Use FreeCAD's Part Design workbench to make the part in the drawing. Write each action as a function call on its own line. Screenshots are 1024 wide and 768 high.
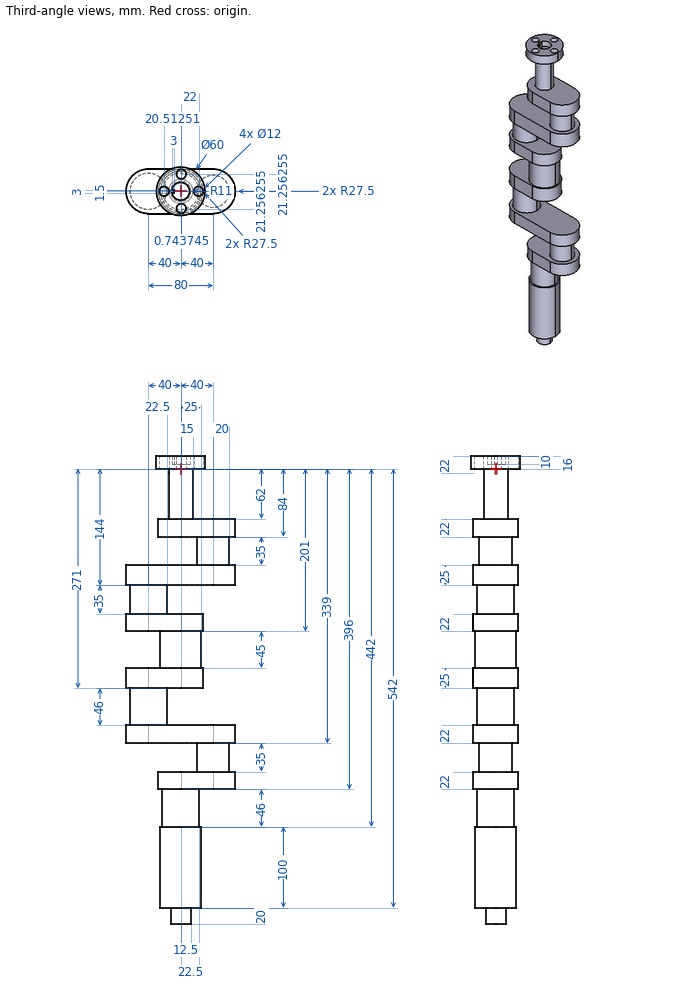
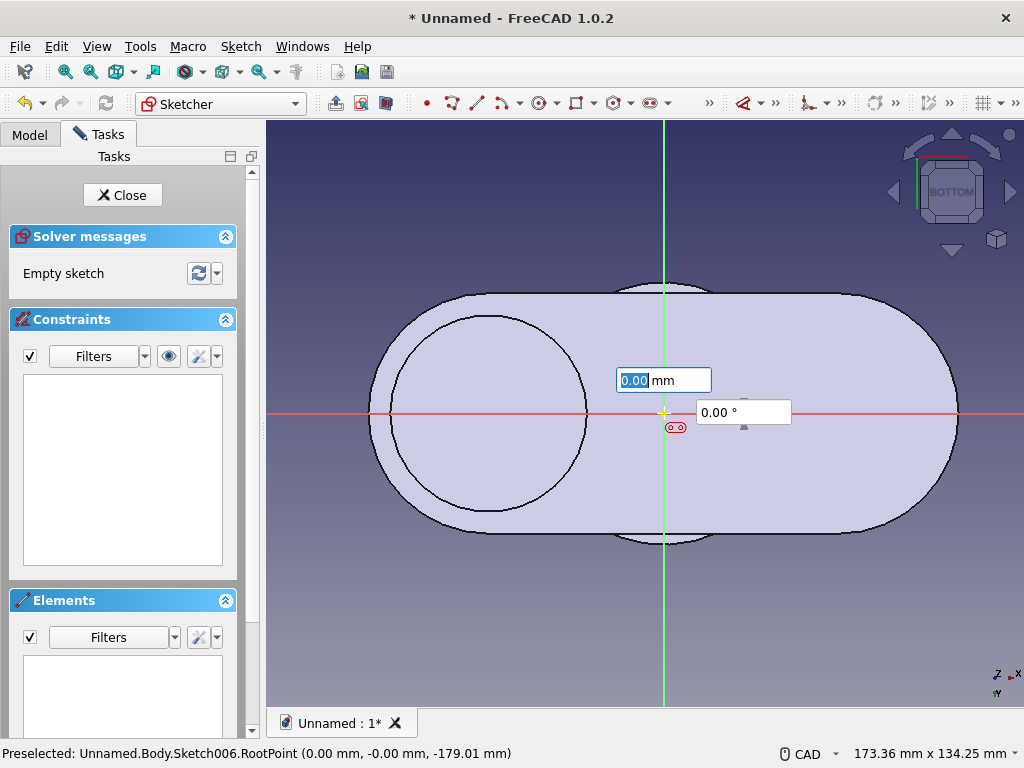
click(489, 404)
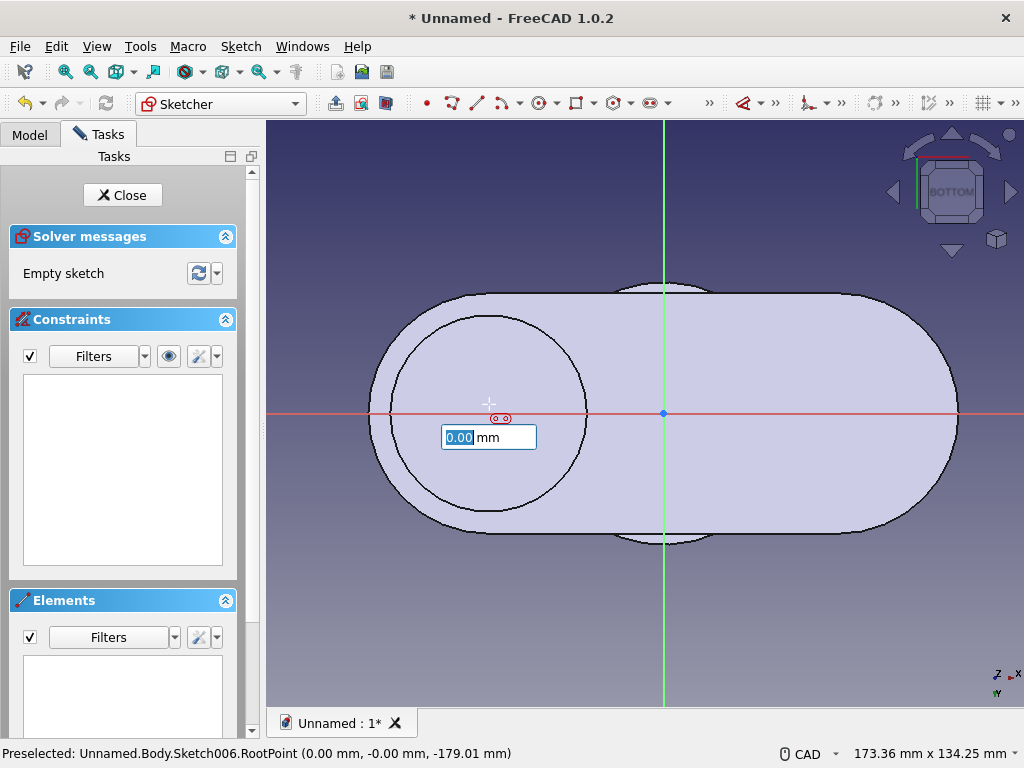
click(576, 534)
key(Escape)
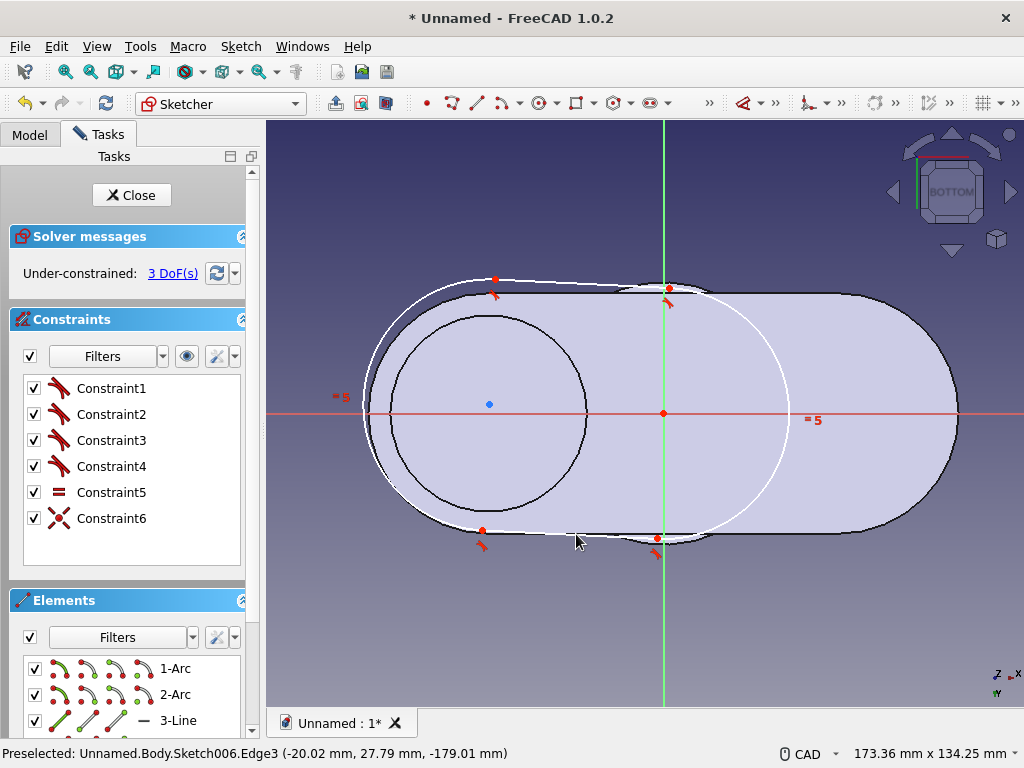
click(605, 536)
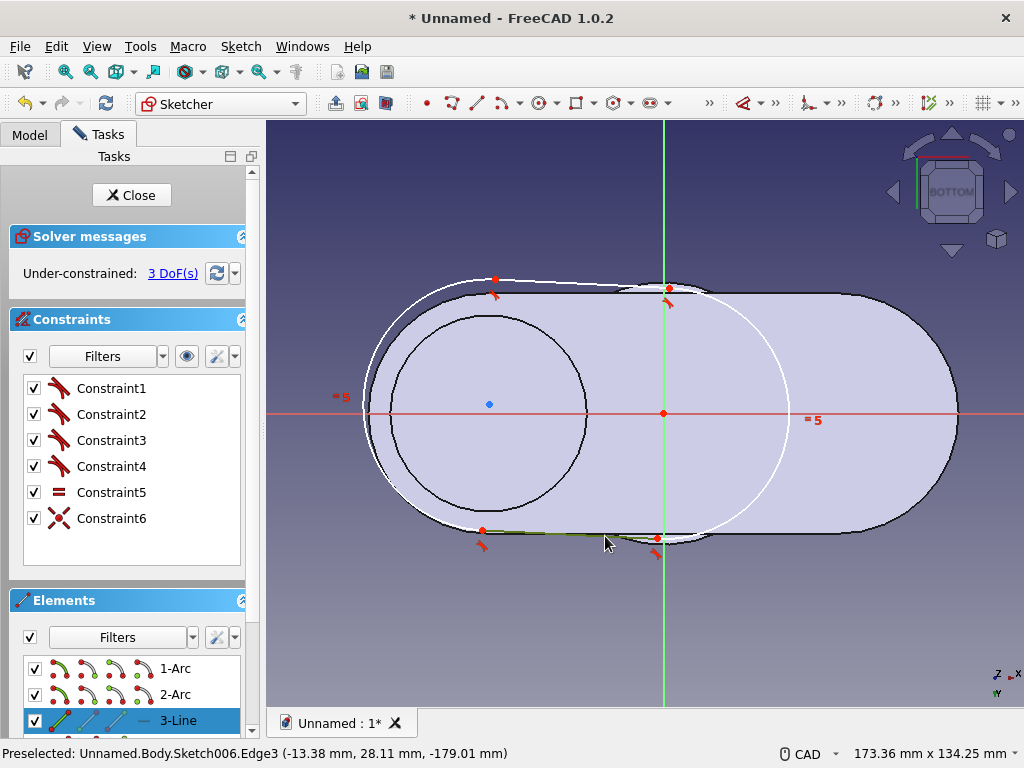
key(h)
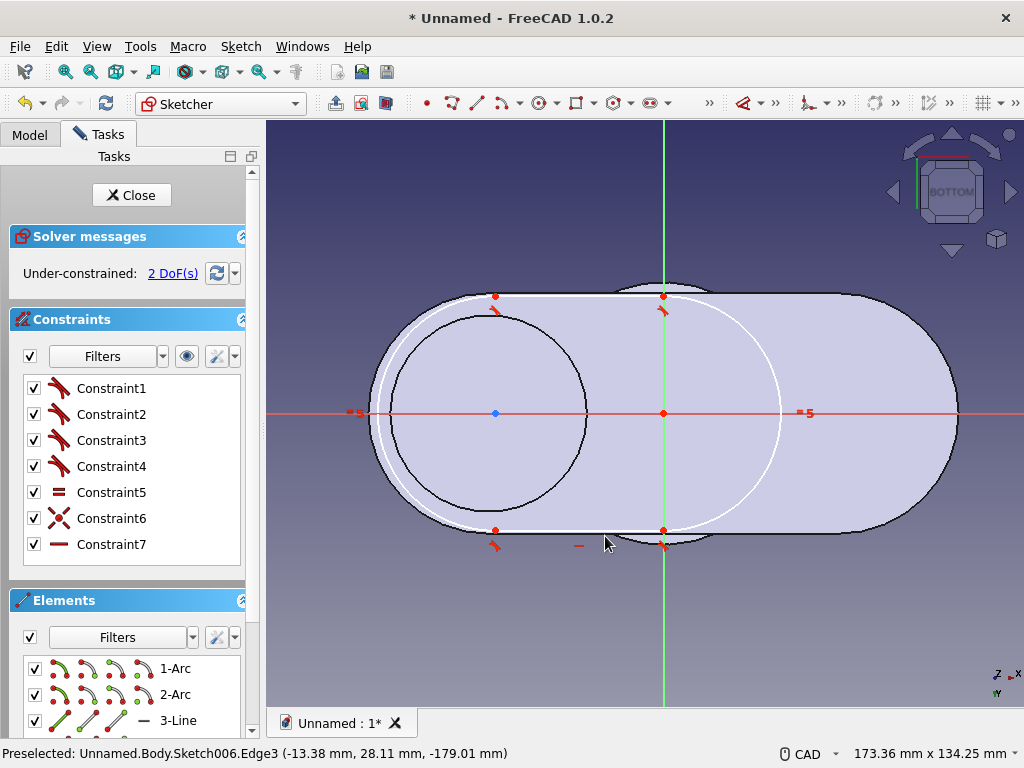
click(742, 104)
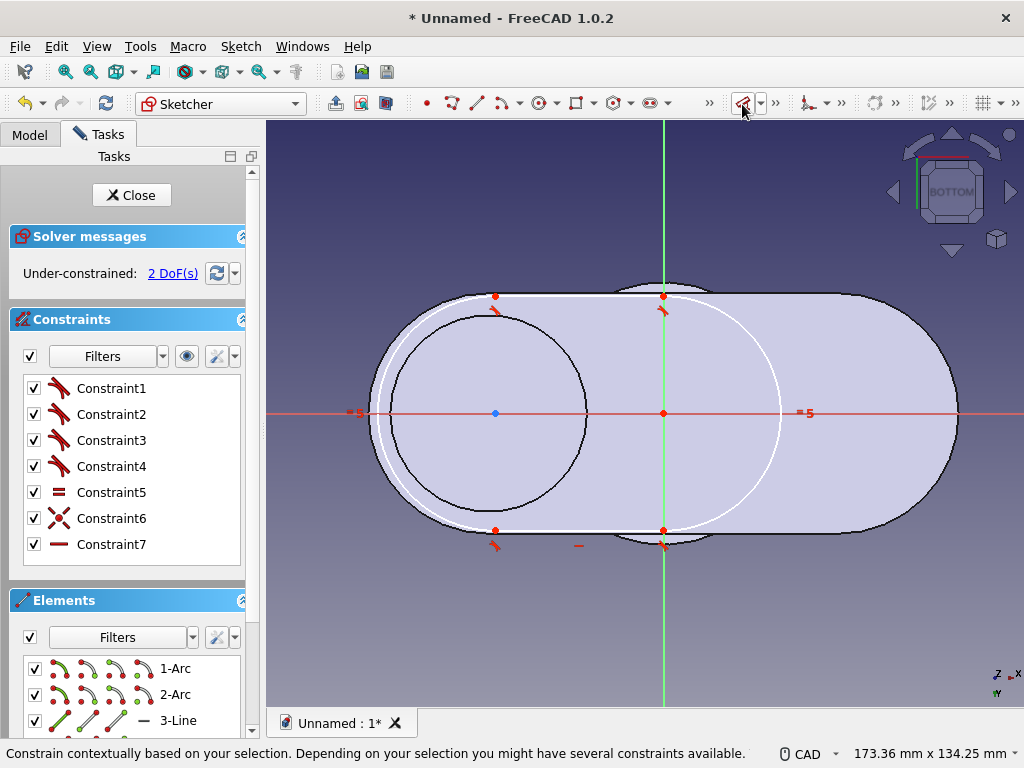
click(758, 482)
click(784, 501)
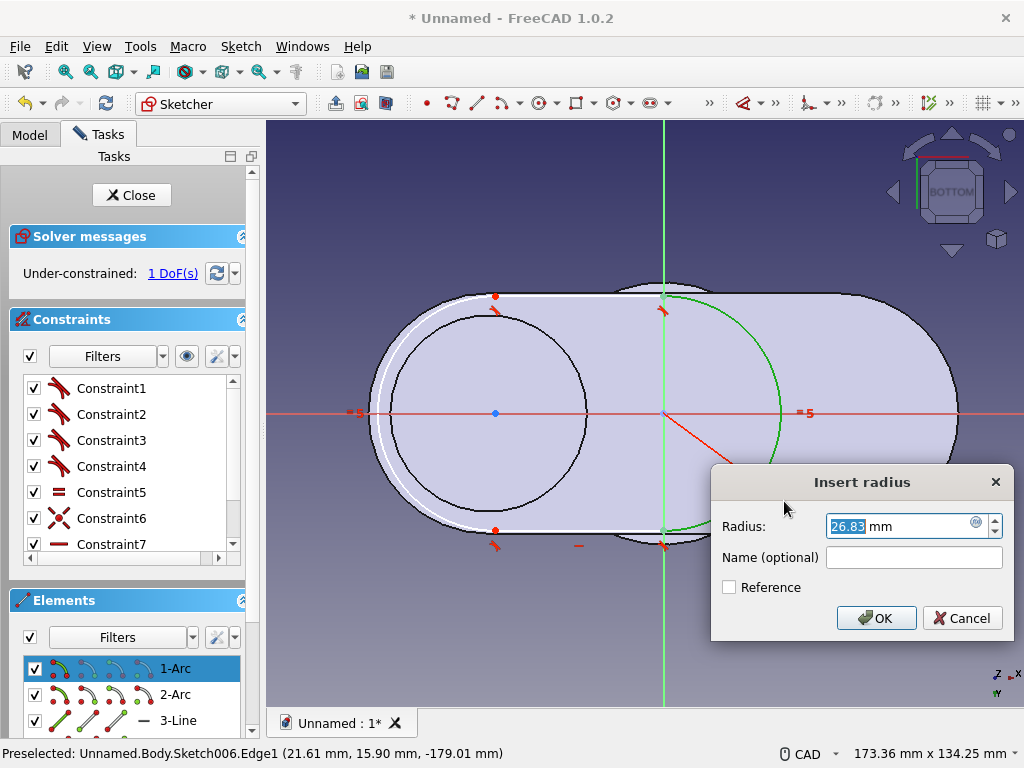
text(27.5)
key(Return)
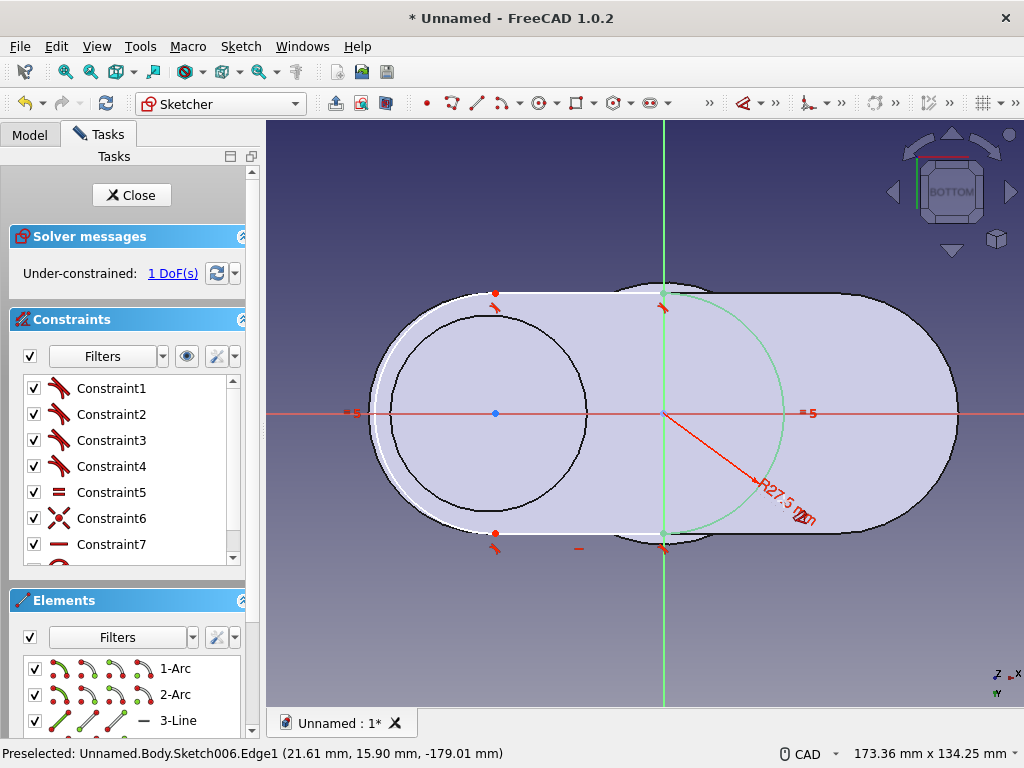
click(613, 534)
click(579, 568)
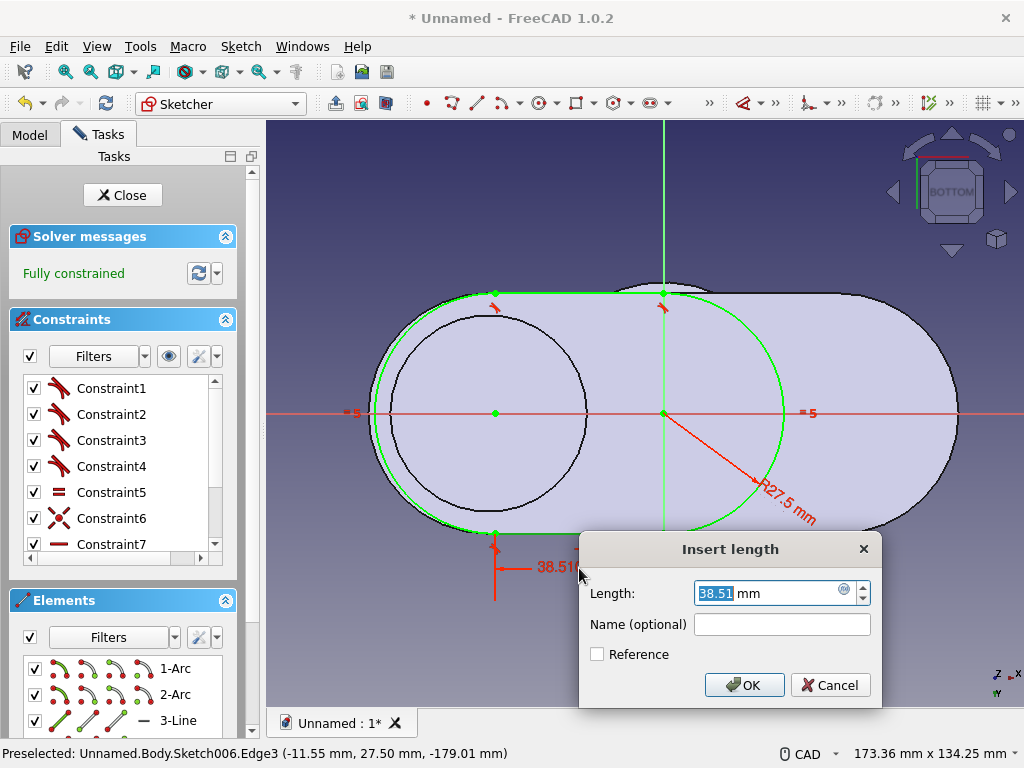
text(40)
key(Return)
key(Escape)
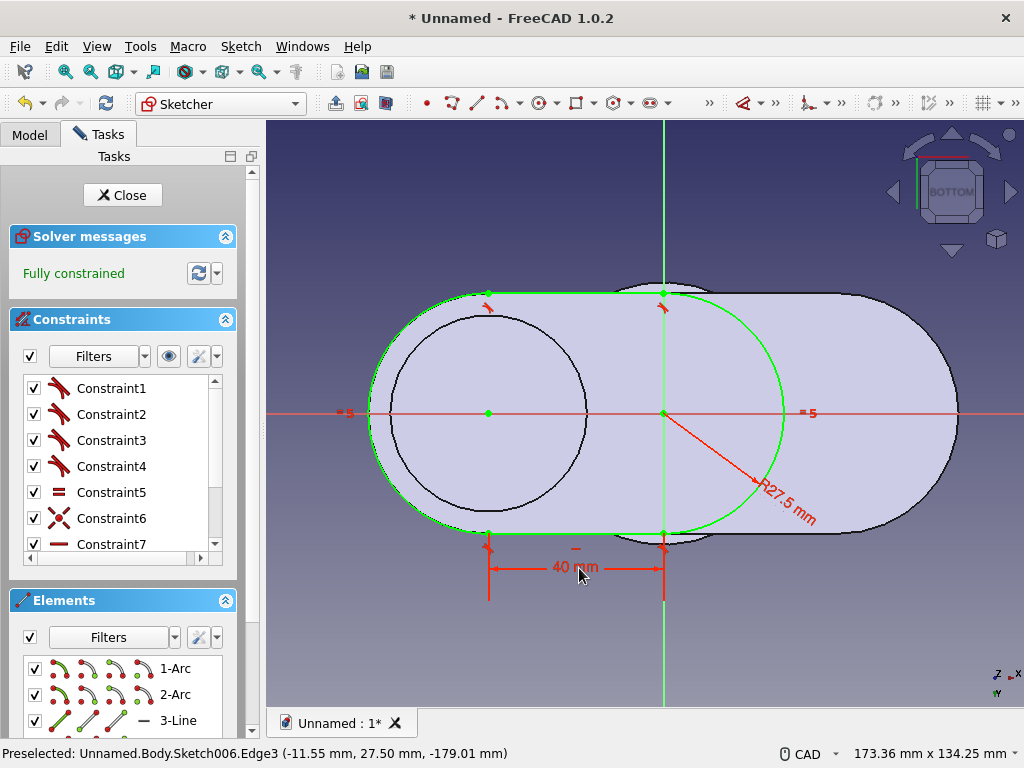
click(123, 195)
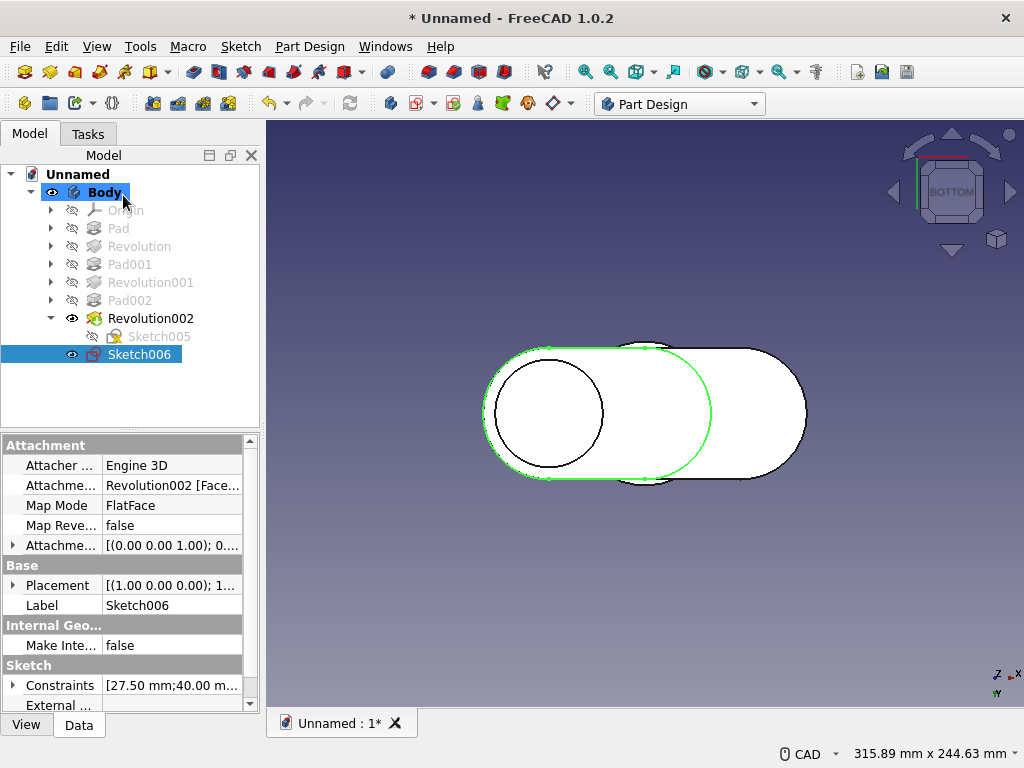
click(25, 72)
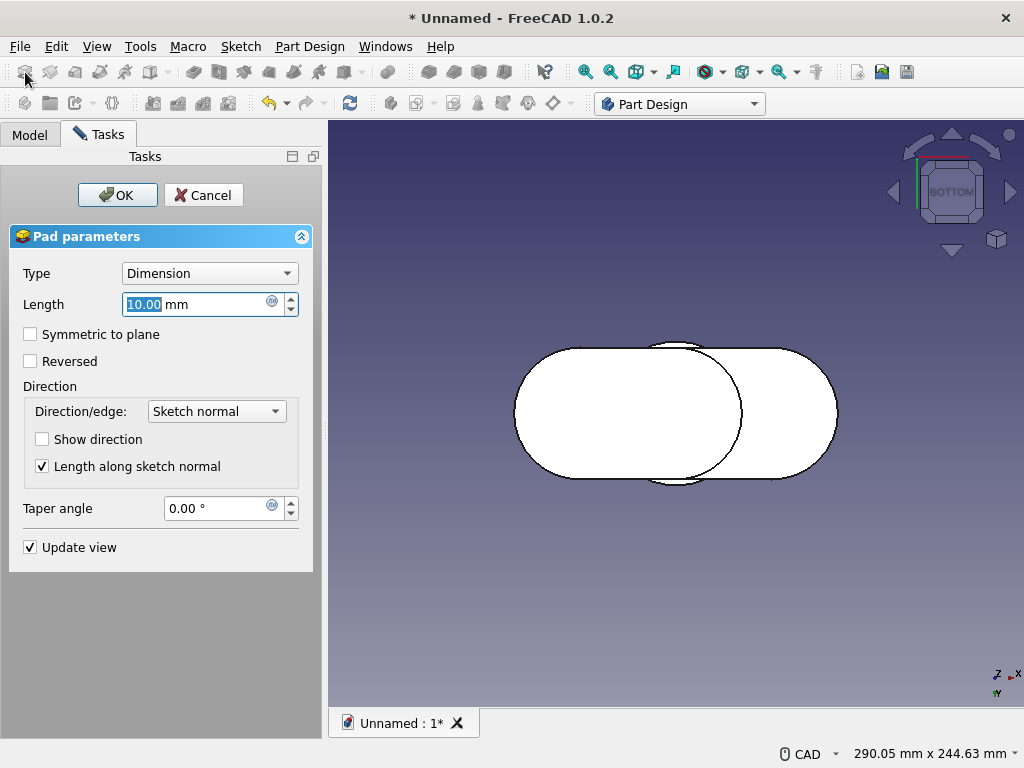
text(22)
key(Tab)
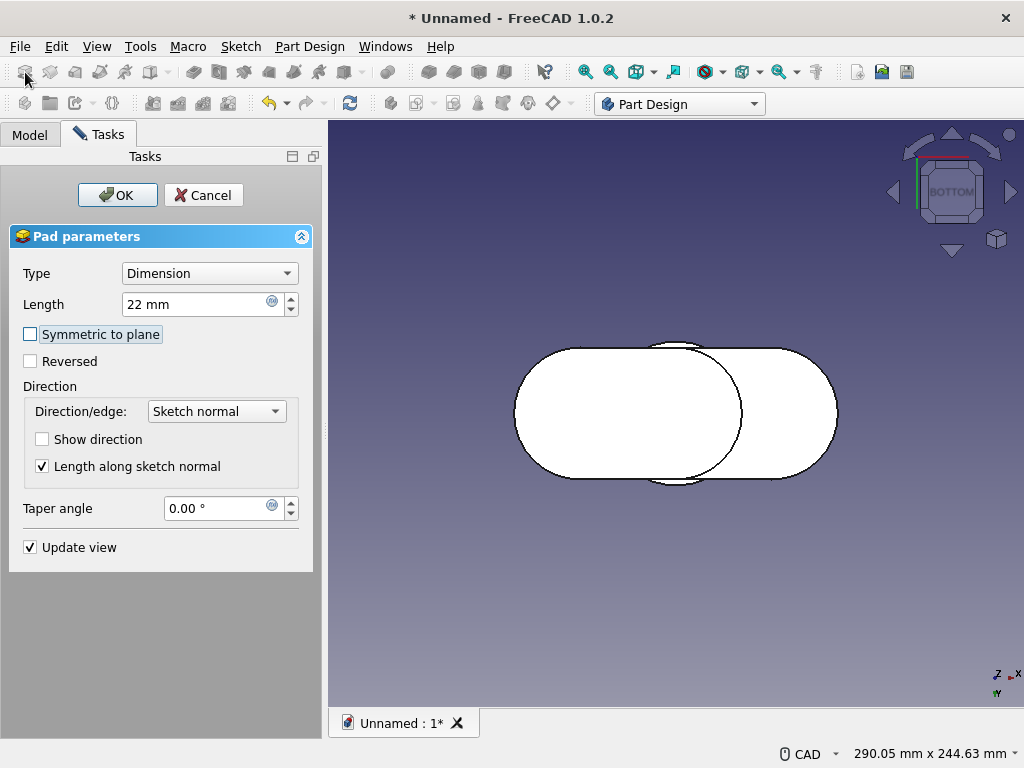
click(118, 195)